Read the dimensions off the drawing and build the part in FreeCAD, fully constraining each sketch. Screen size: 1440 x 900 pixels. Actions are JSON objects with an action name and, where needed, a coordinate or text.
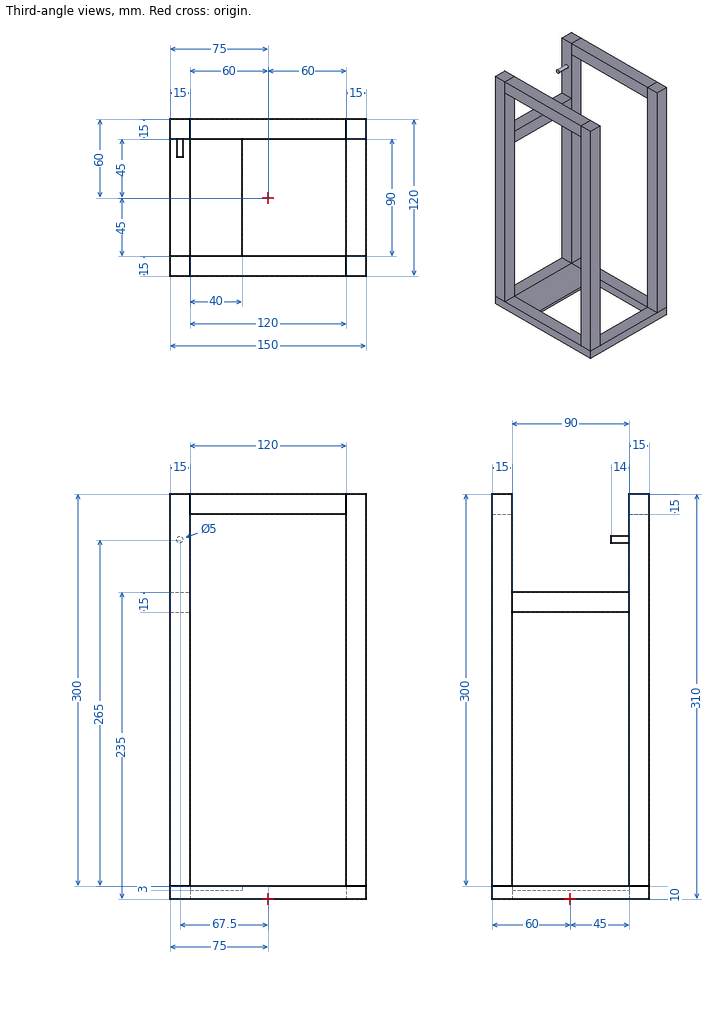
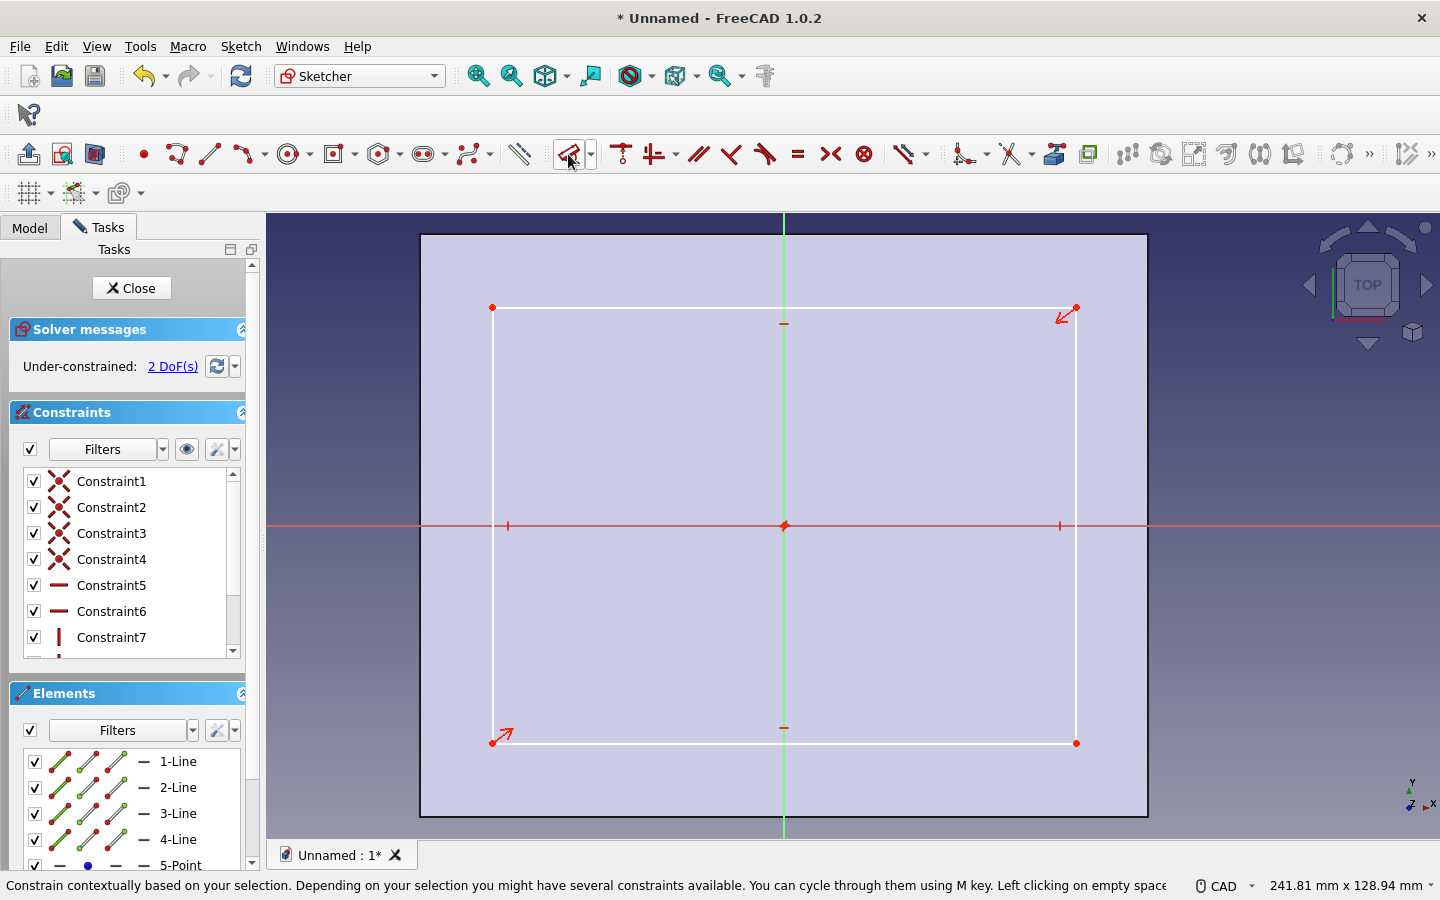
{"action": "left_click", "coordinate": [1076, 613]}
{"action": "left_click", "coordinate": [1110, 426]}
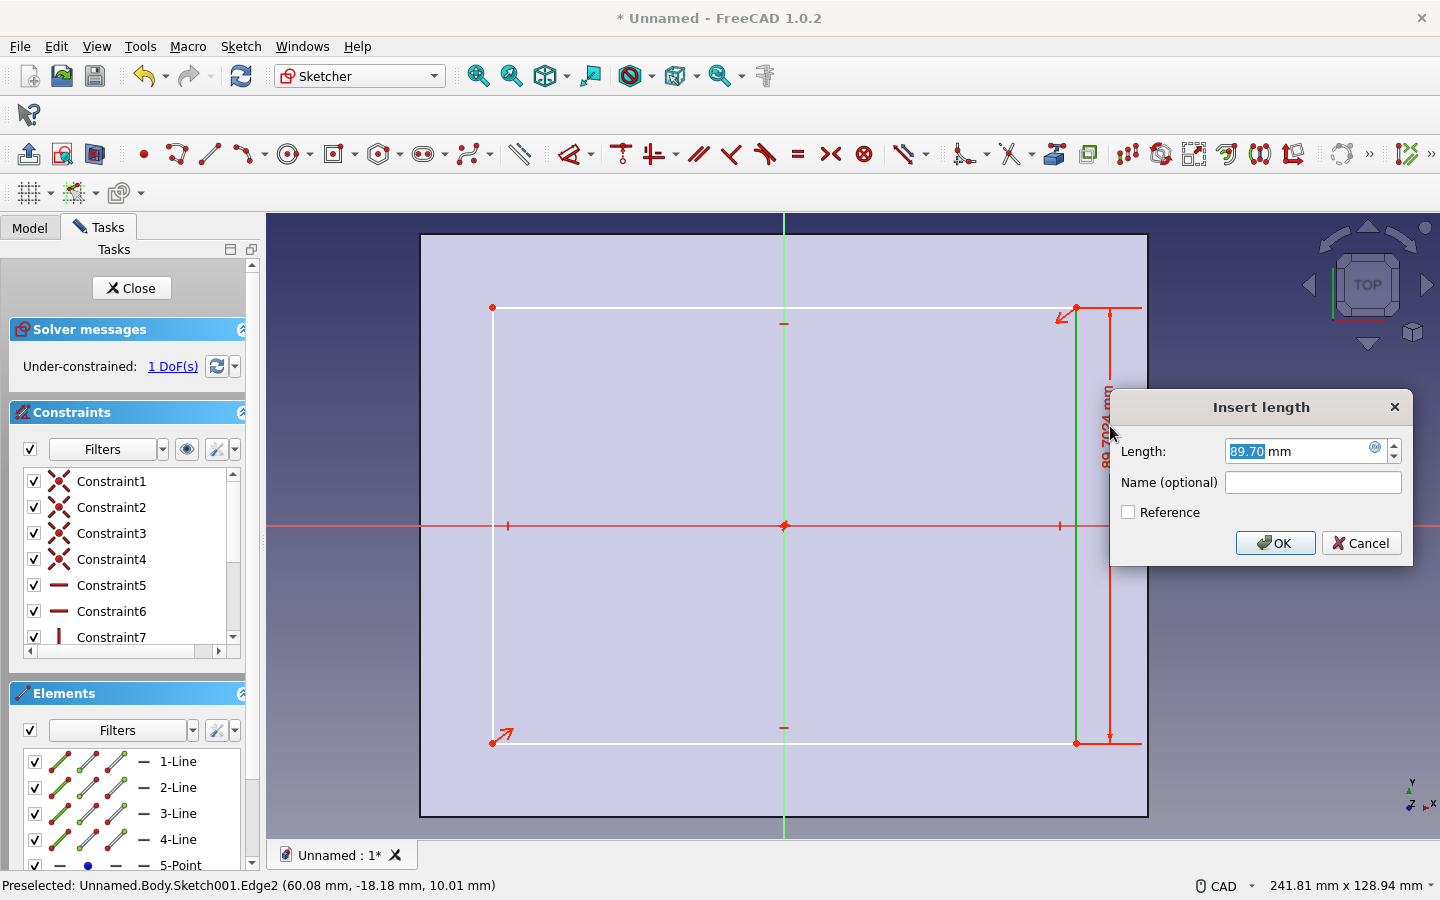
{"action": "type", "text": "90"}
{"action": "key", "text": "Return"}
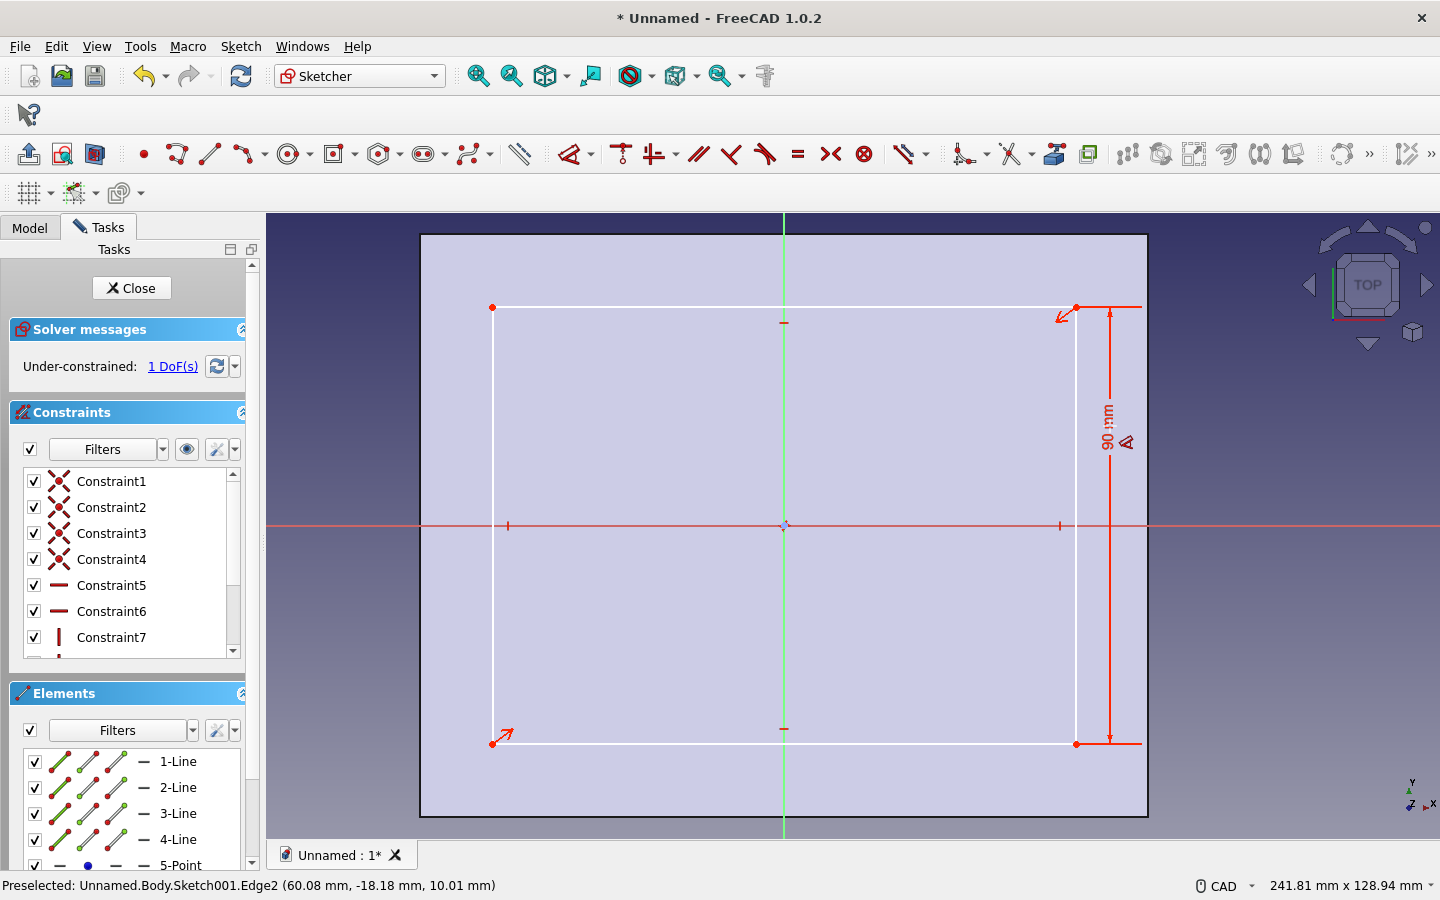
{"action": "left_click", "coordinate": [668, 744]}
{"action": "left_click", "coordinate": [650, 778]}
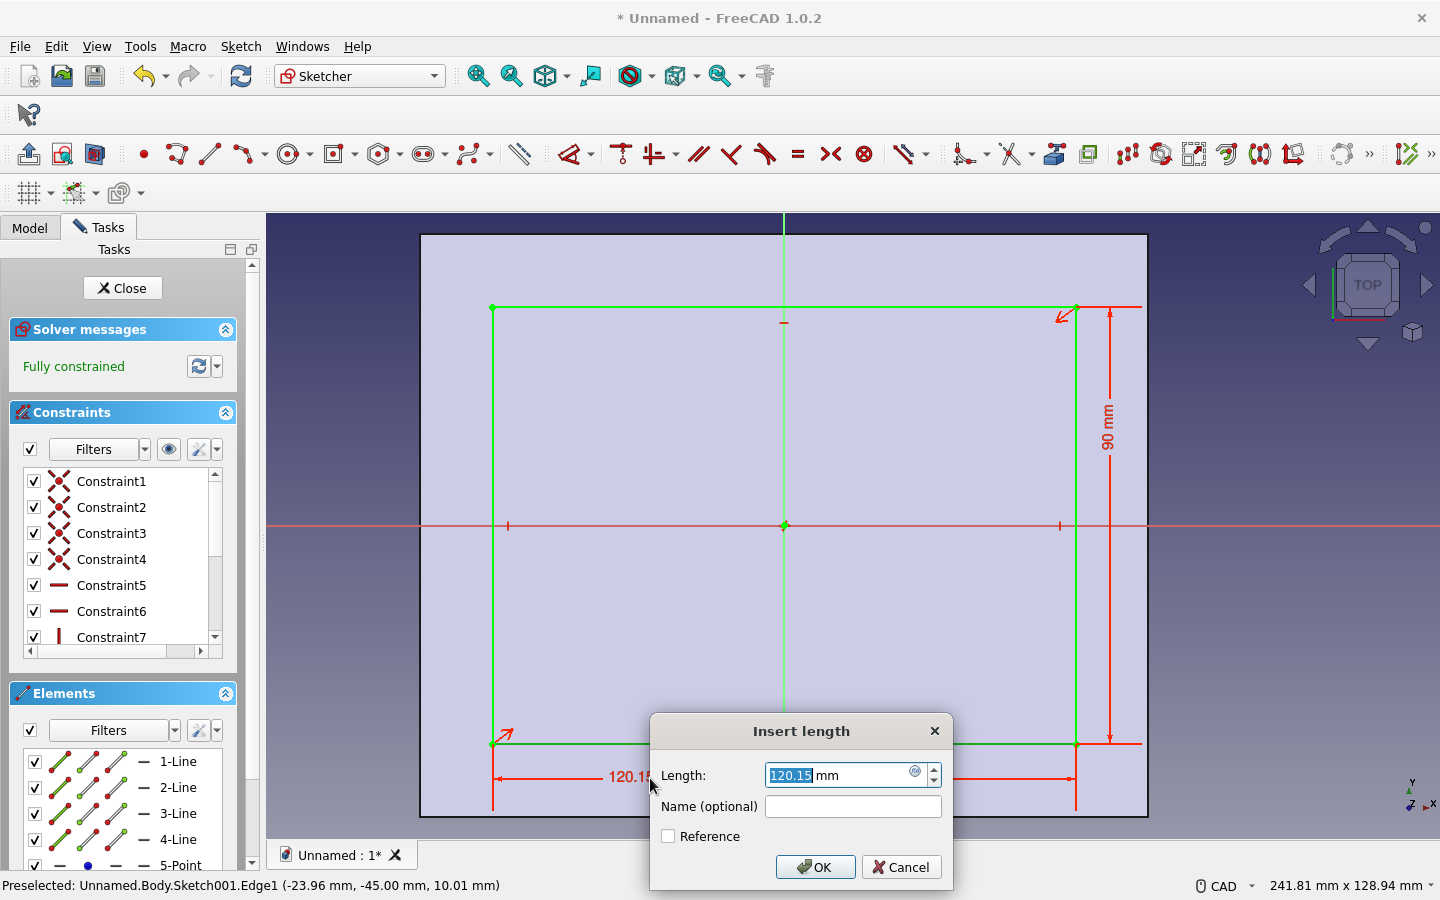
{"action": "type", "text": "120"}
{"action": "key", "text": "Return"}
{"action": "key", "text": "Escape"}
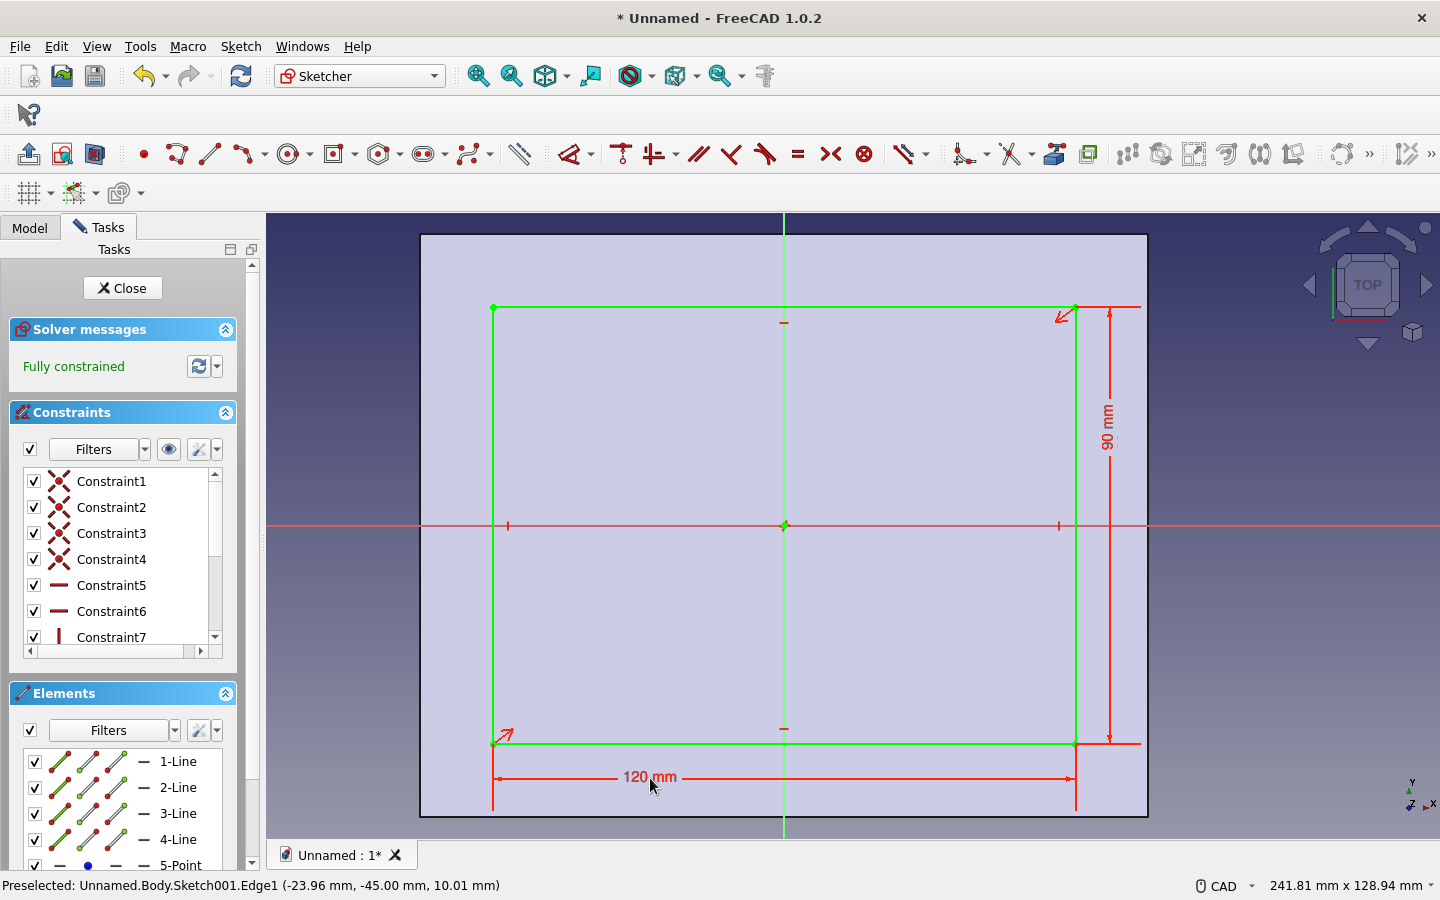
{"action": "left_click", "coordinate": [123, 288]}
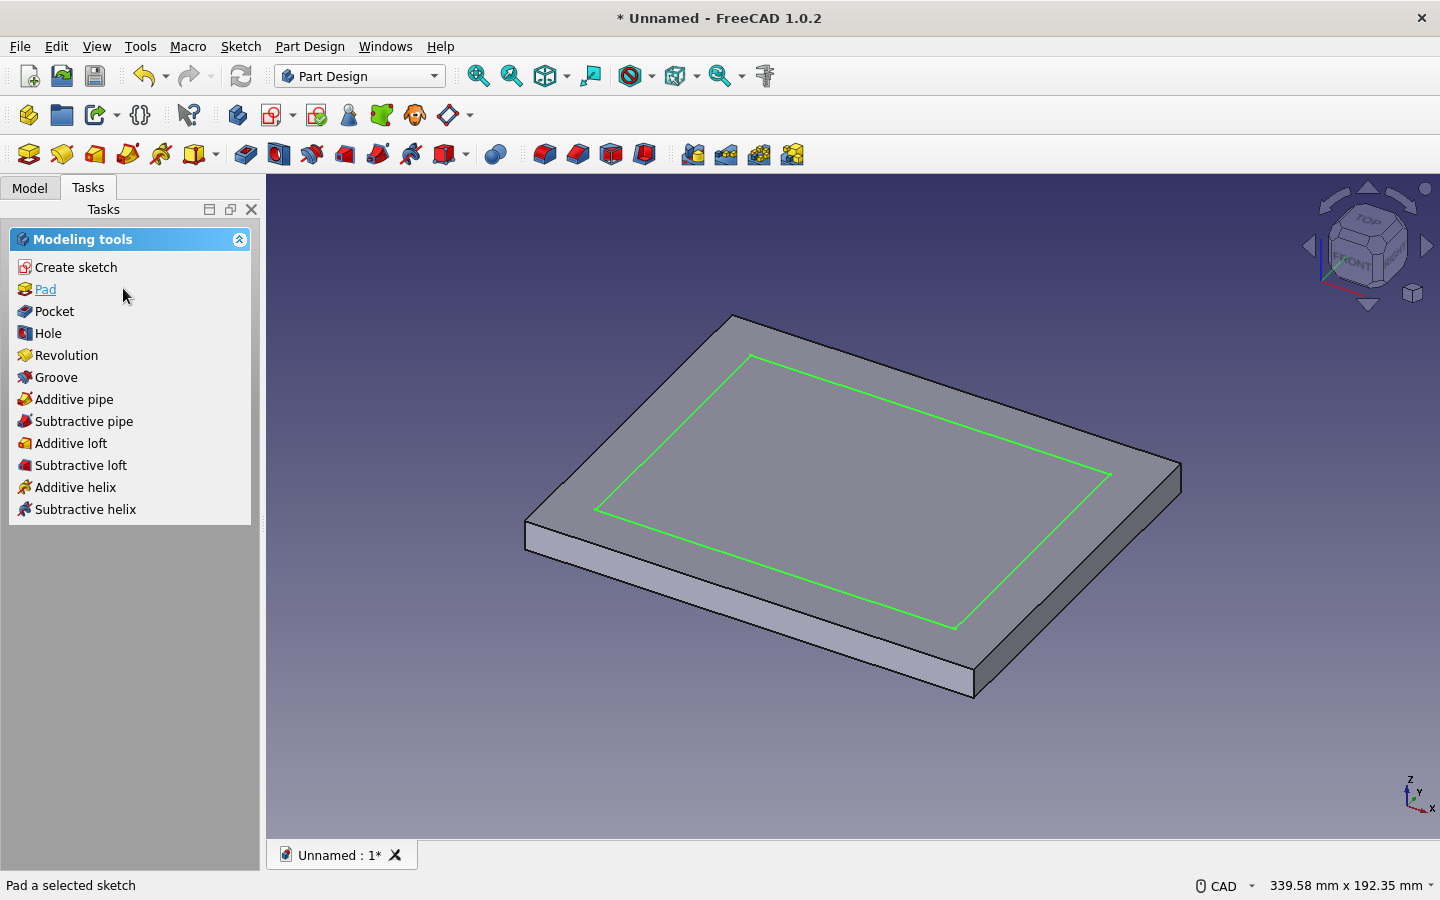
{"action": "left_click", "coordinate": [246, 154]}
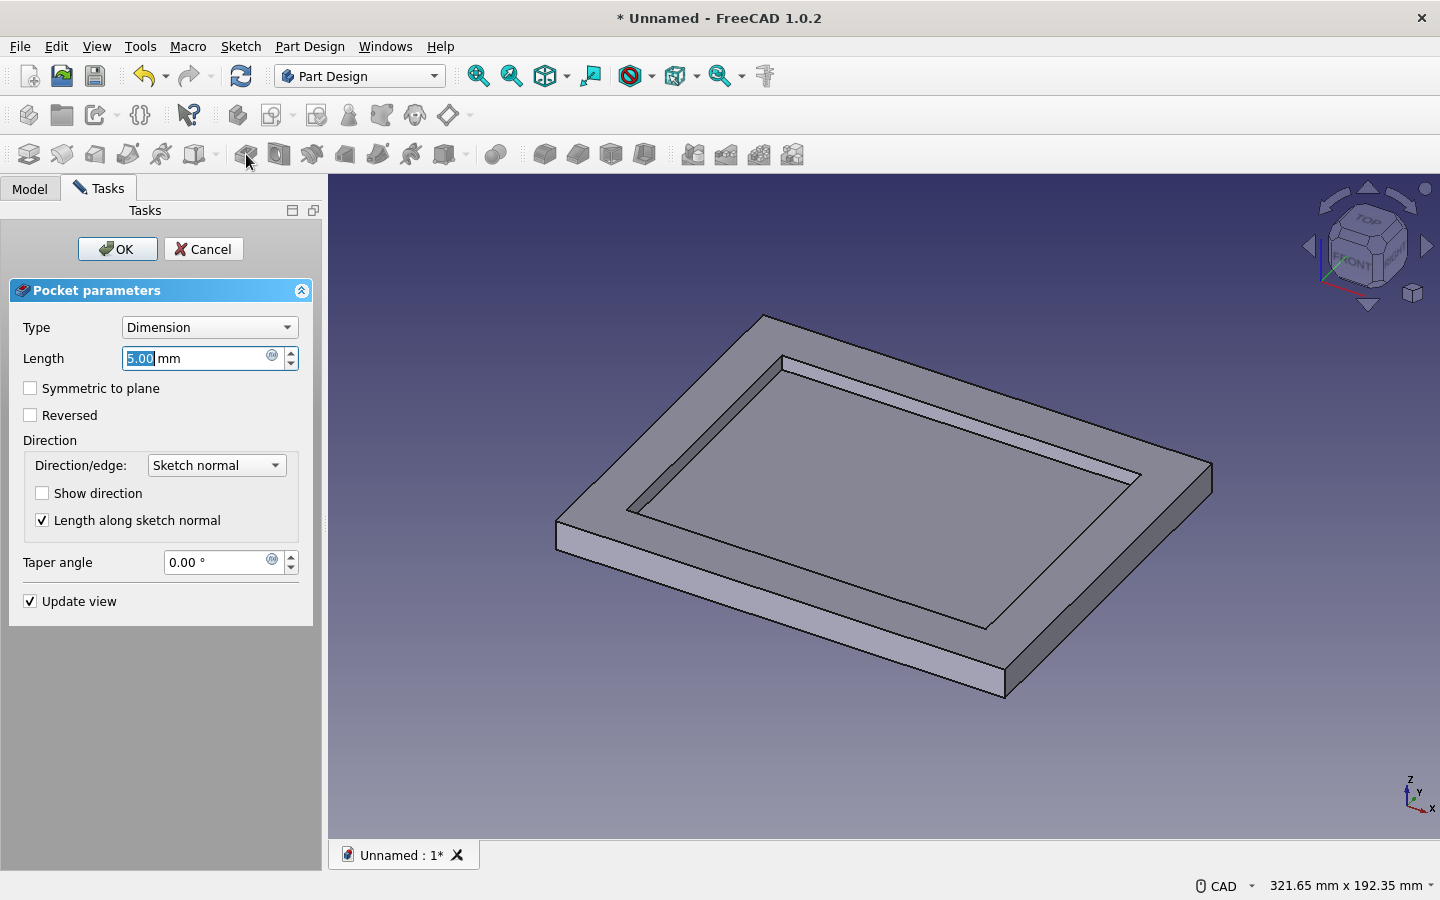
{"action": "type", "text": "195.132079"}
{"action": "key", "text": "Tab"}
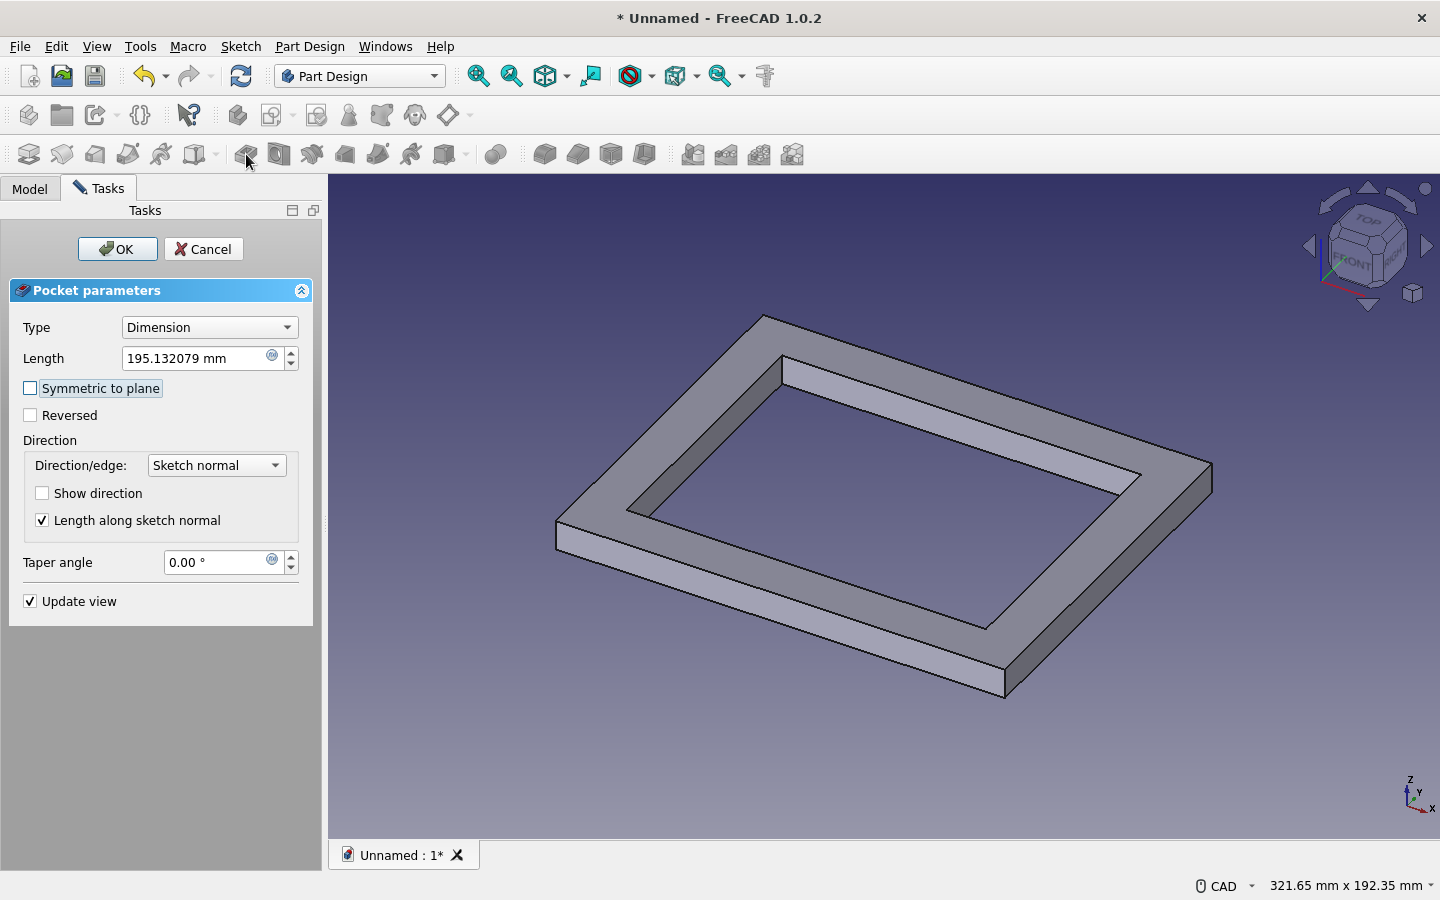
{"action": "left_click", "coordinate": [31, 388]}